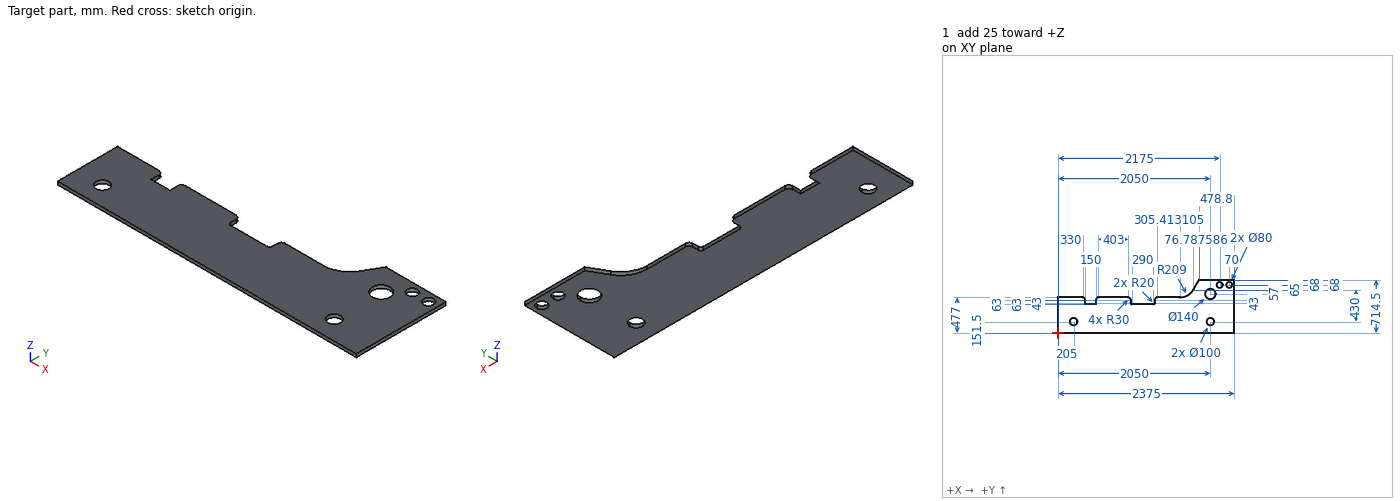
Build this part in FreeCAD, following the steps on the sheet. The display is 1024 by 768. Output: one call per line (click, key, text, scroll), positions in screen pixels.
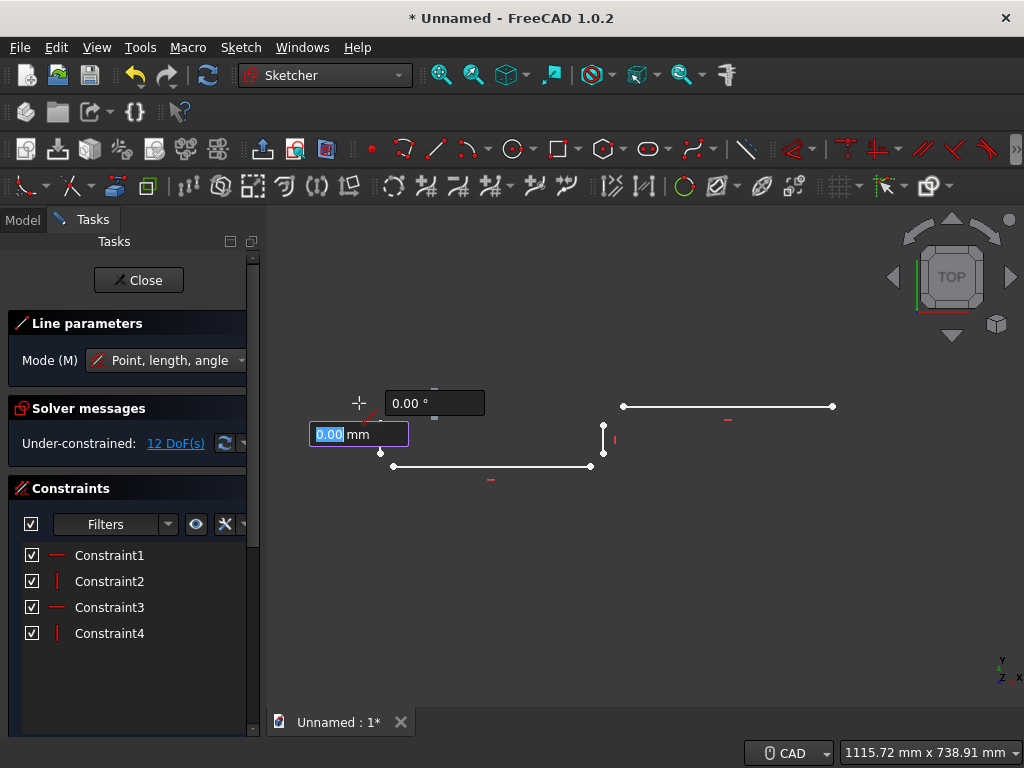
scroll(593, 447, down, 7)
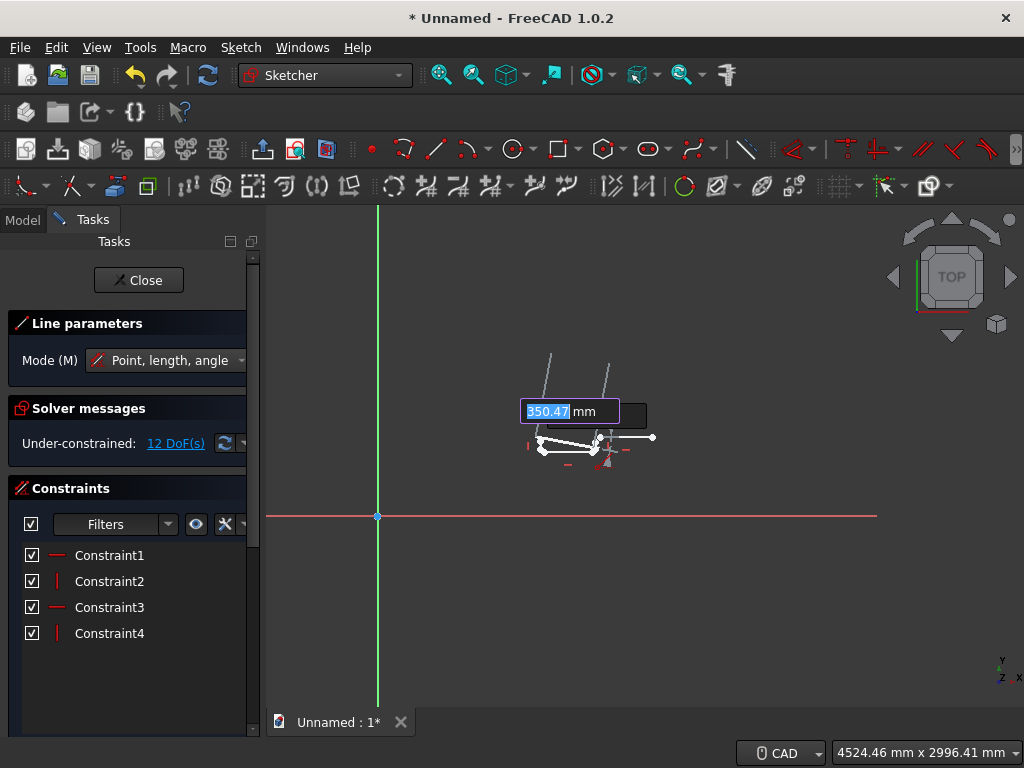
click(468, 437)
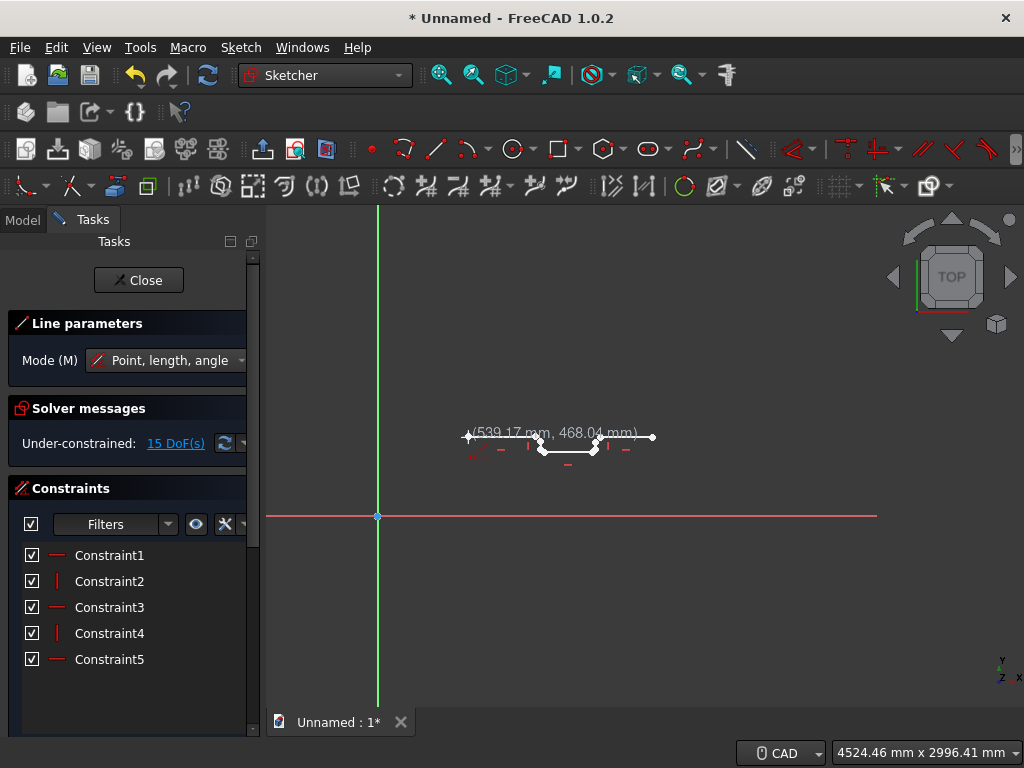
click(404, 150)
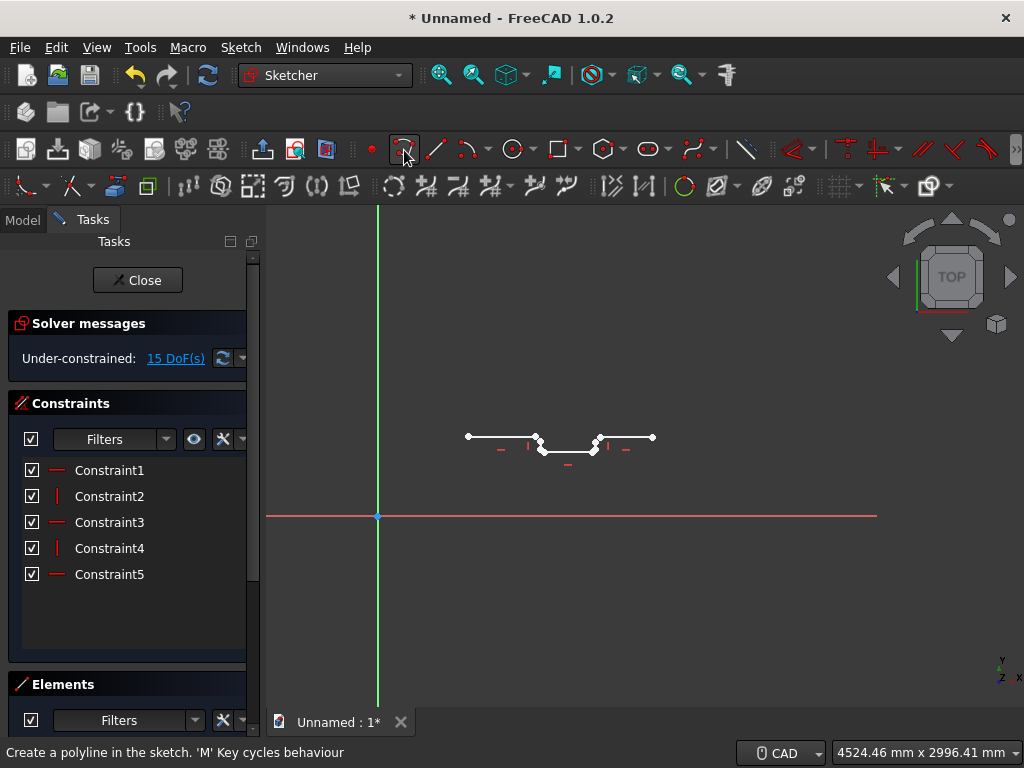
scroll(463, 442, up, 5)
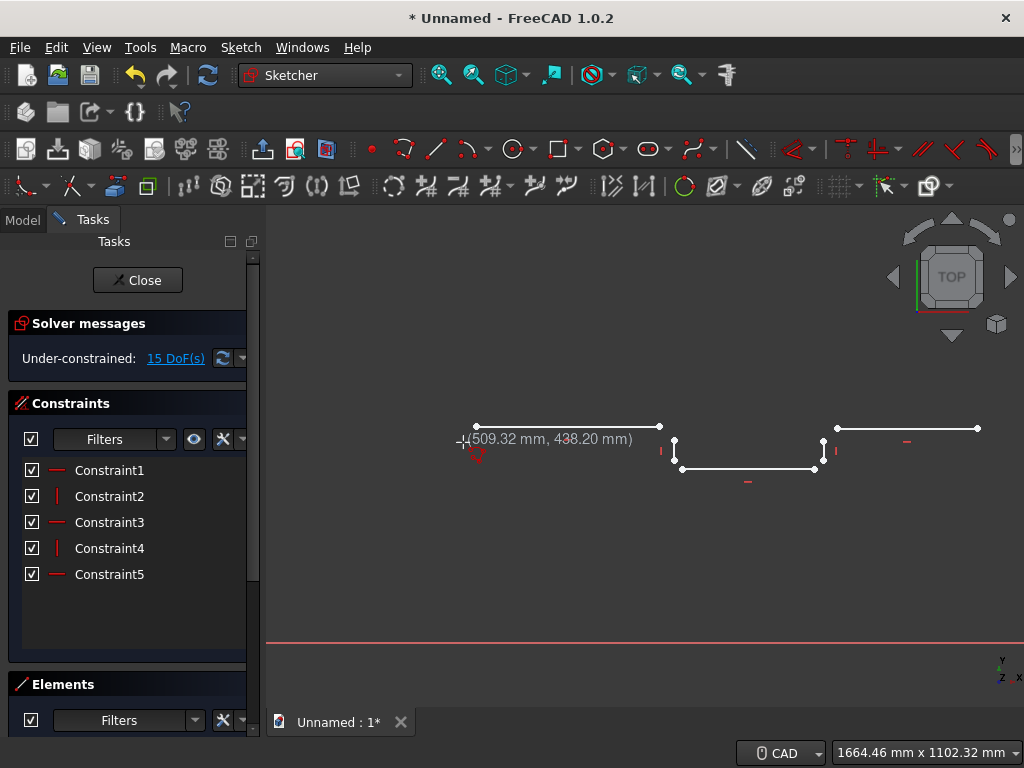
click(463, 440)
click(463, 469)
click(395, 469)
click(395, 440)
right_click(395, 440)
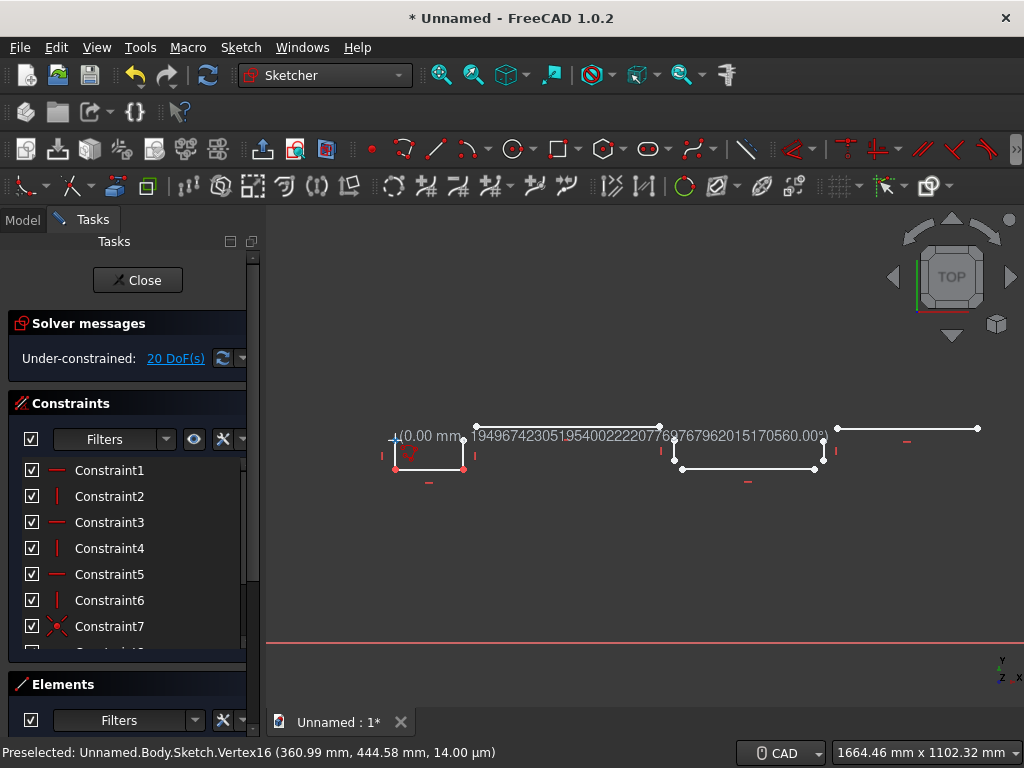
click(381, 426)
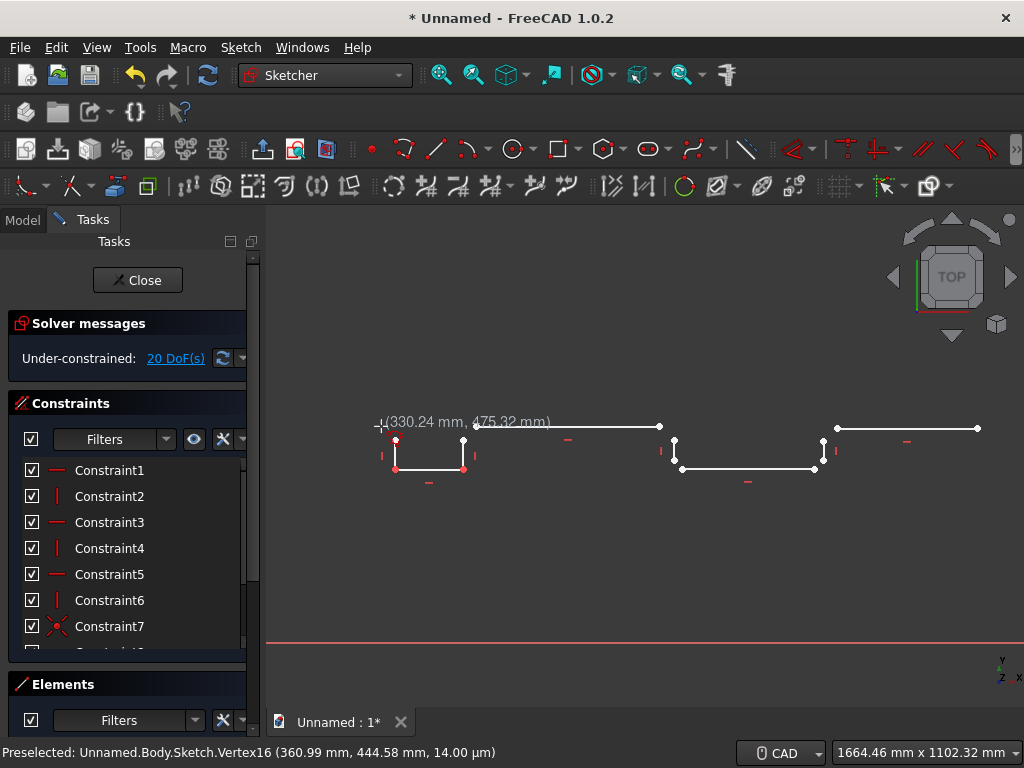
scroll(463, 442, down, 5)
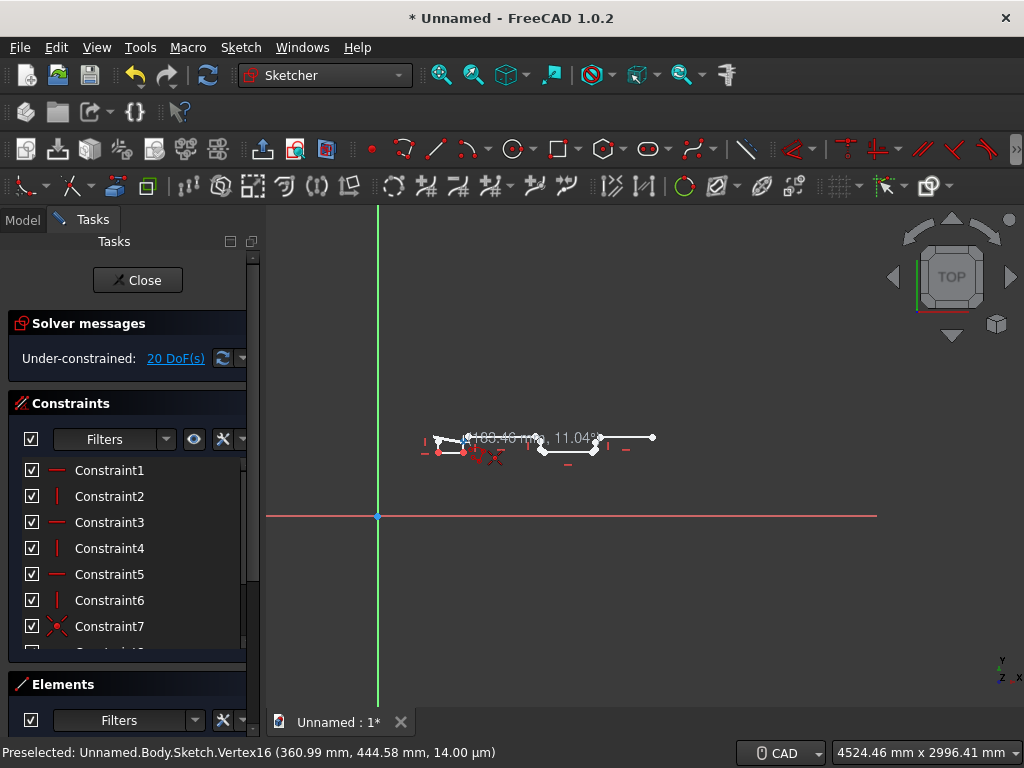
click(378, 436)
click(378, 516)
click(776, 507)
click(776, 397)
click(695, 397)
click(682, 419)
right_click(682, 419)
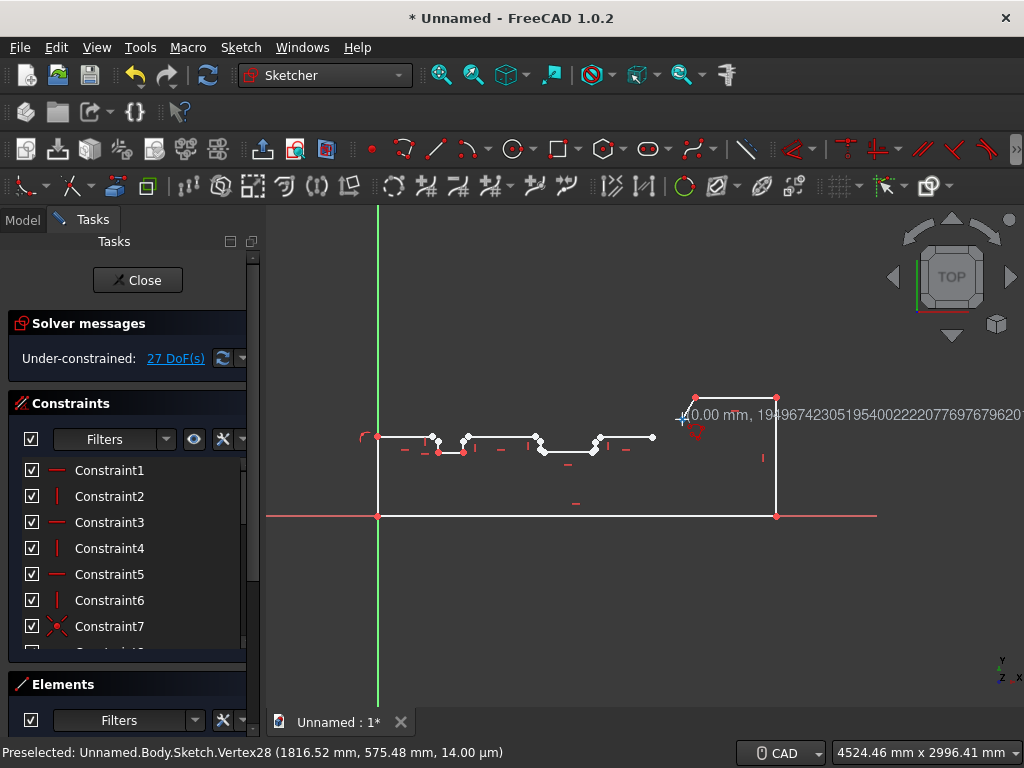
click(490, 150)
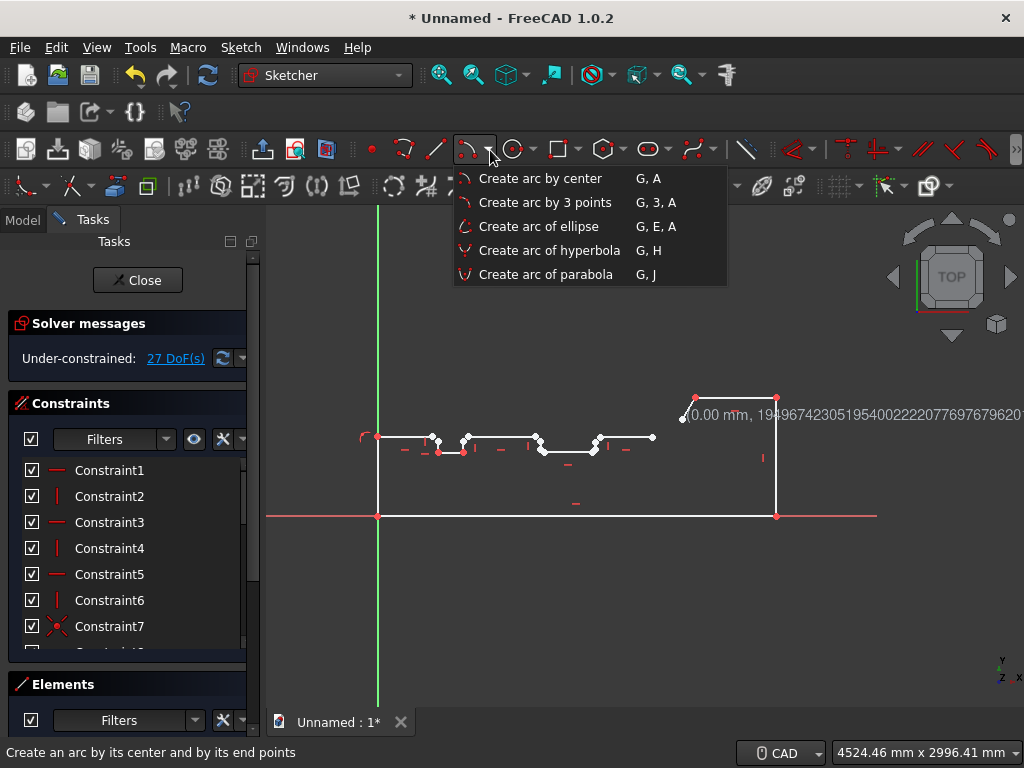
click(590, 202)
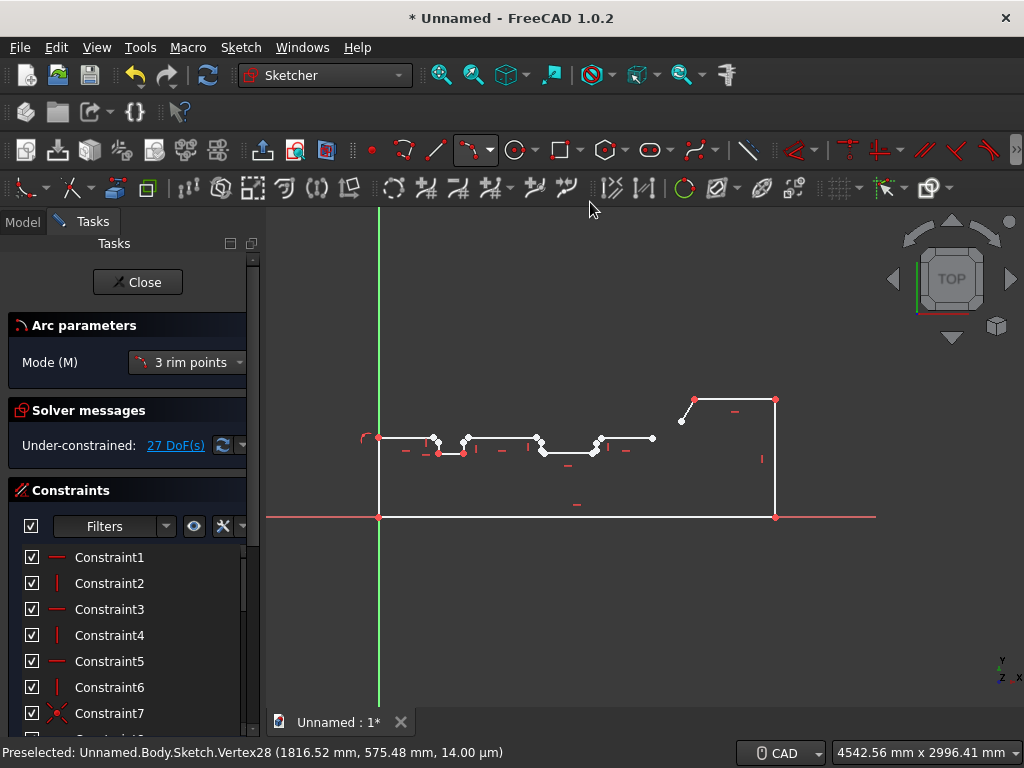
scroll(601, 438, up, 5)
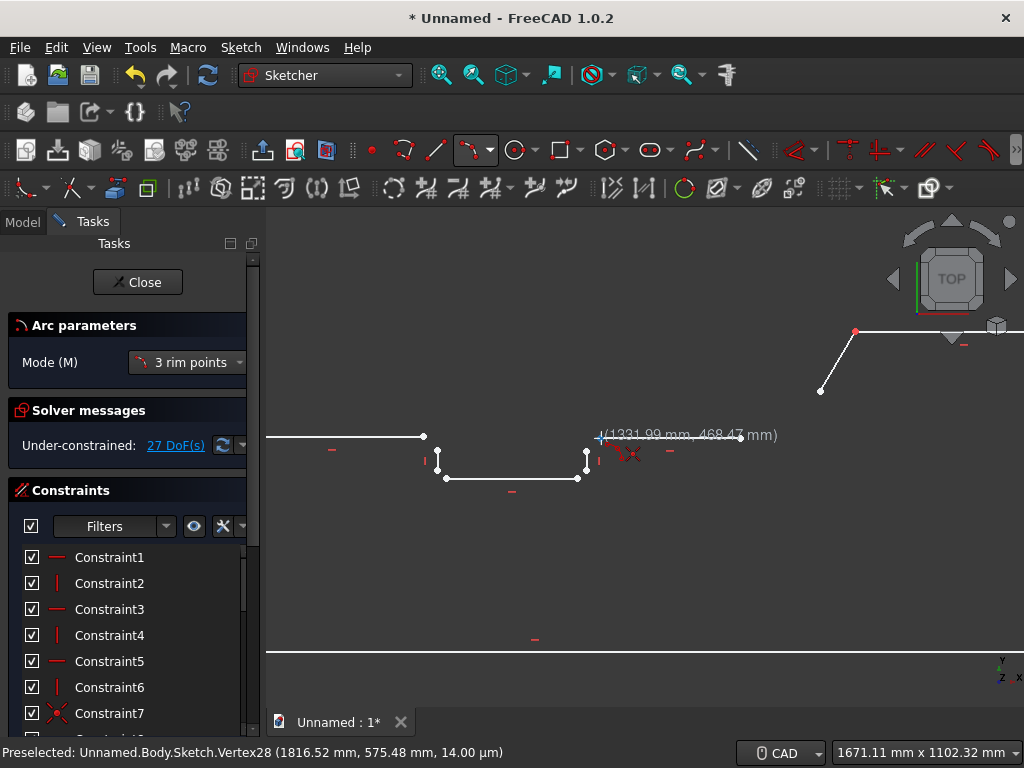
click(601, 438)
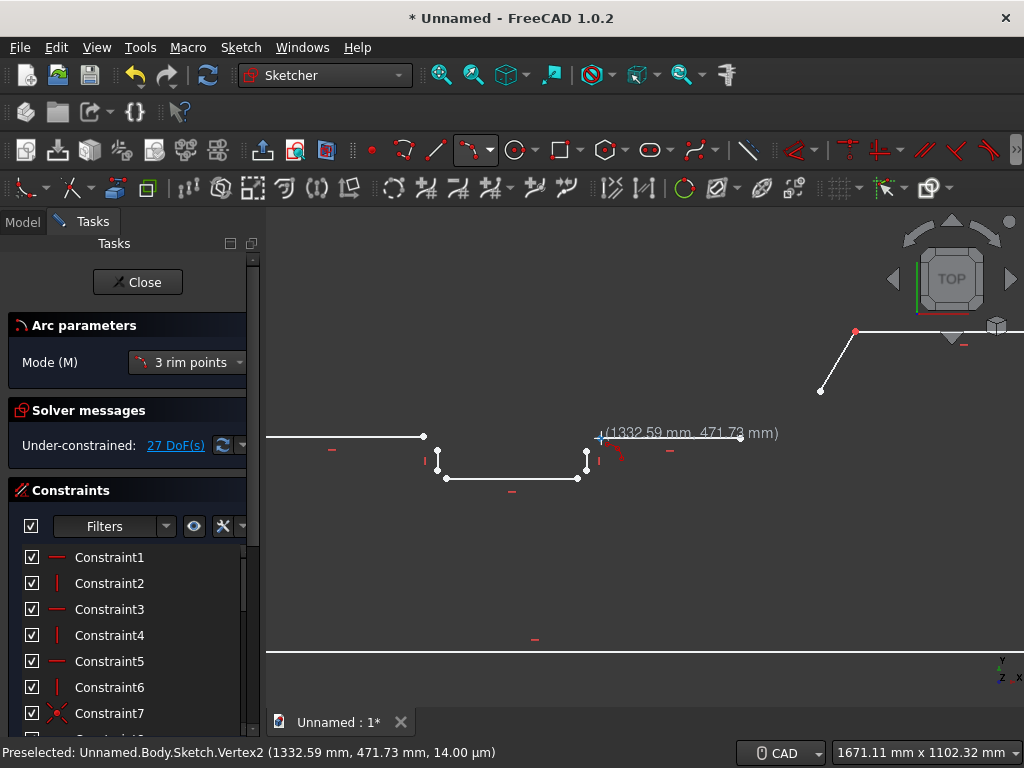
scroll(587, 450, up, 3)